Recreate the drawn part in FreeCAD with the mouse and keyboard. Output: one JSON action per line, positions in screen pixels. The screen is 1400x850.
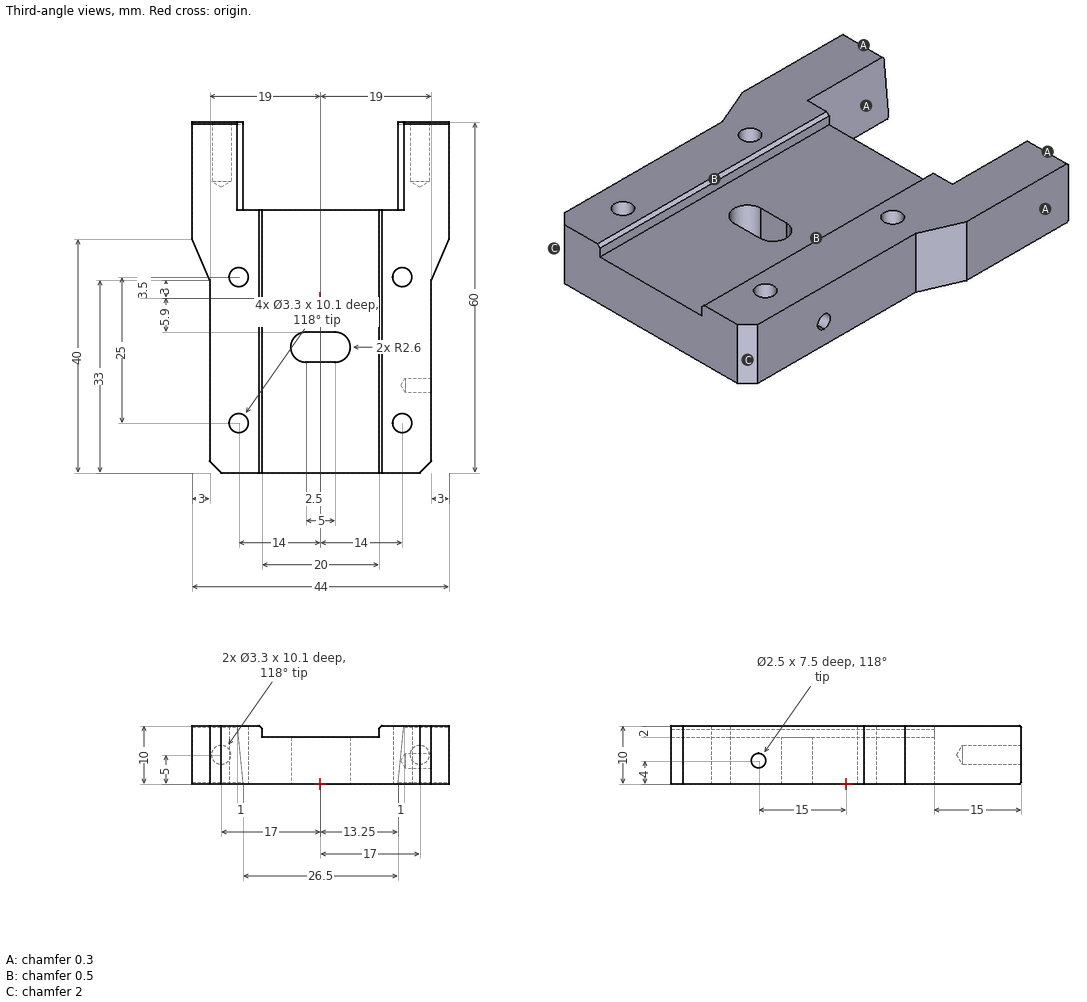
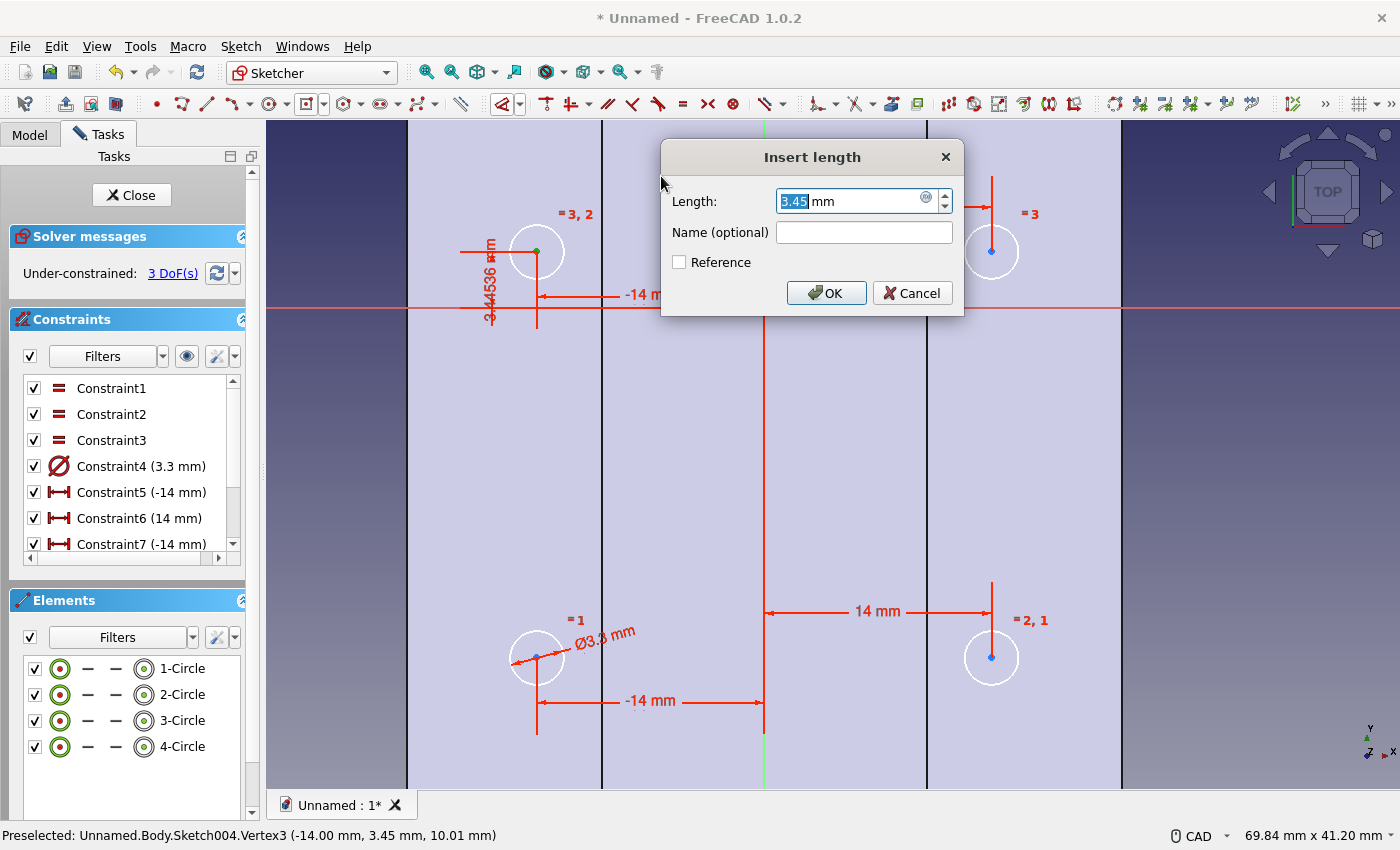
{"action": "type", "text": "3.5"}
{"action": "key", "text": "Return"}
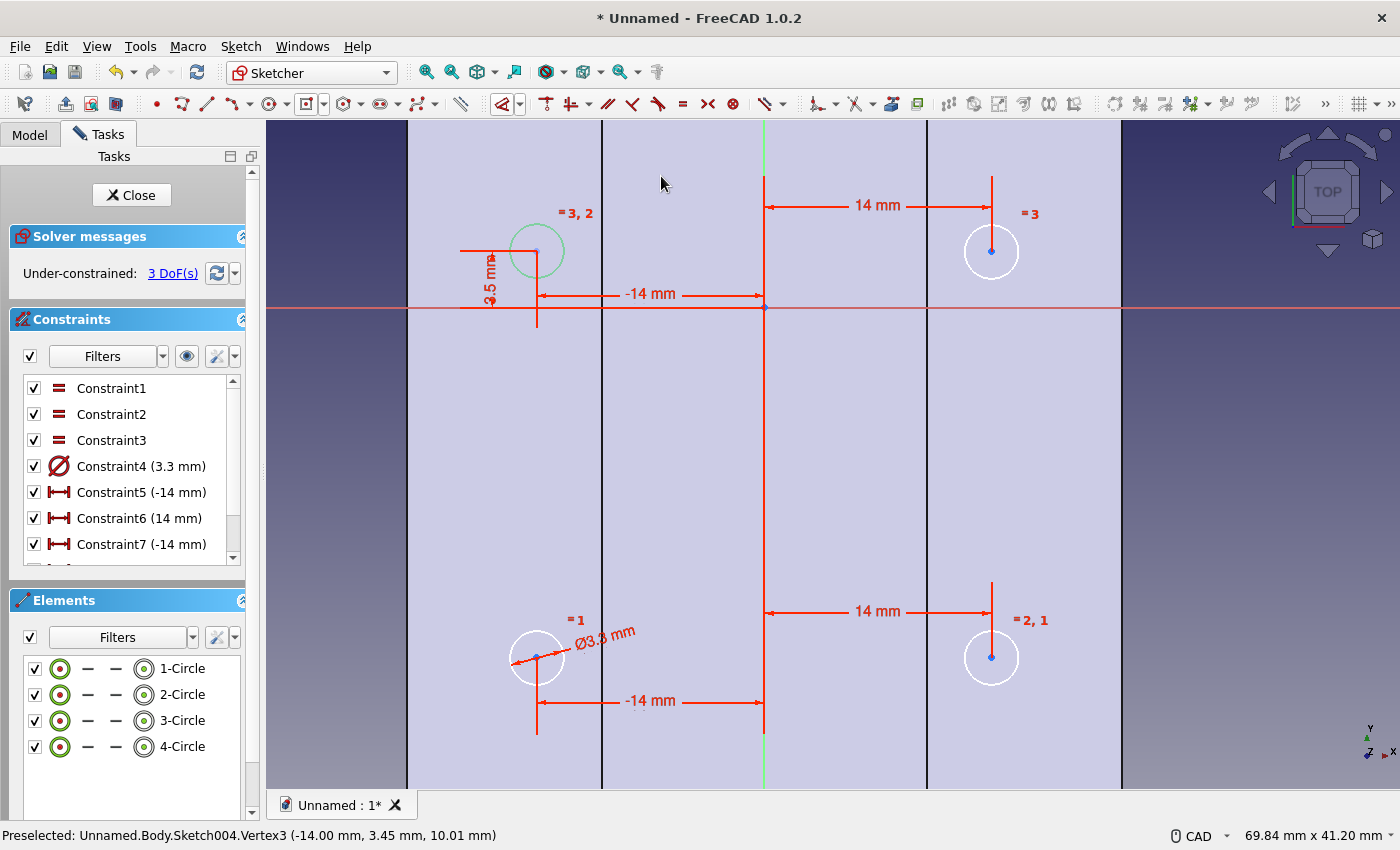
{"action": "left_click", "coordinate": [992, 252]}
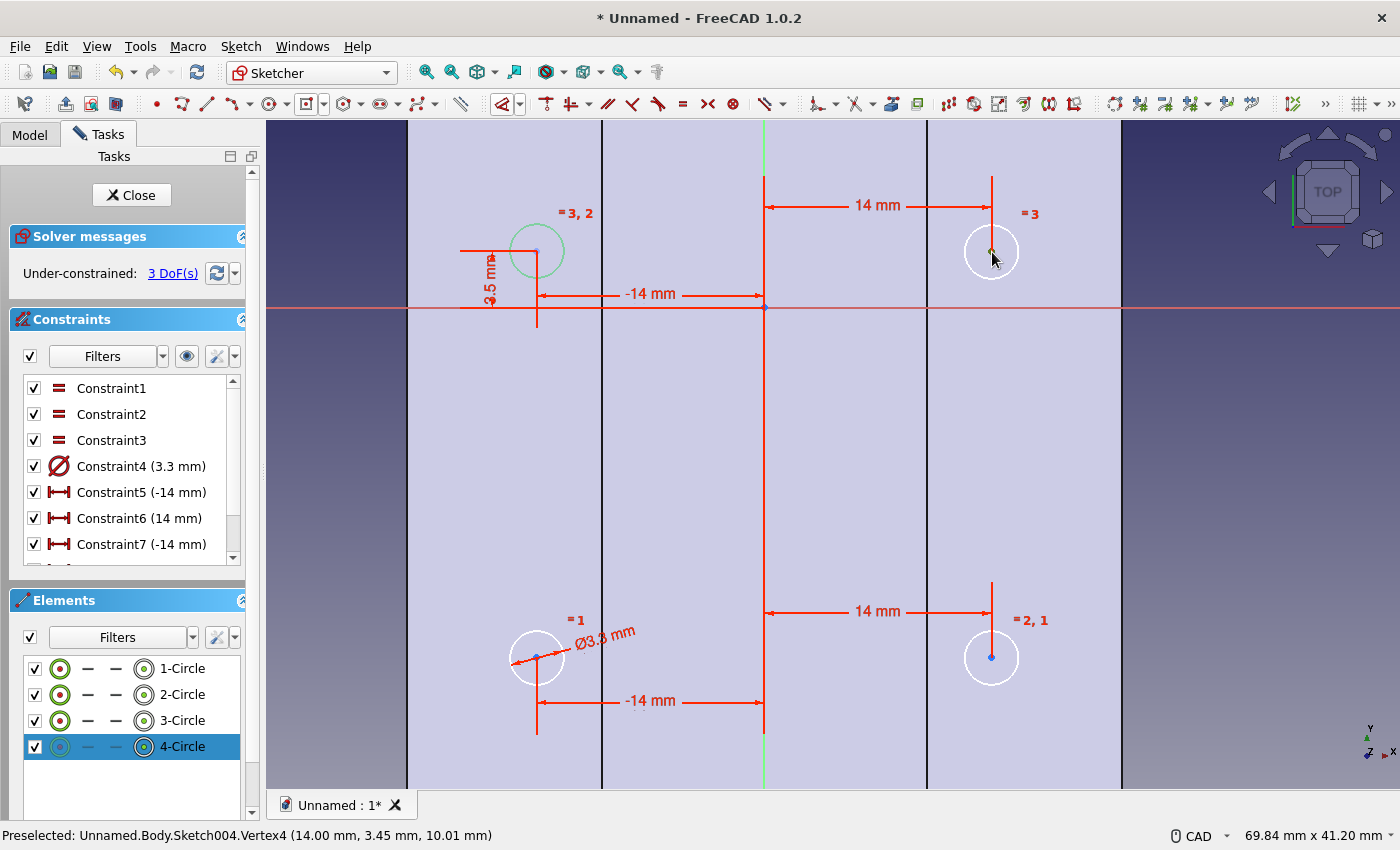
{"action": "key", "text": "i"}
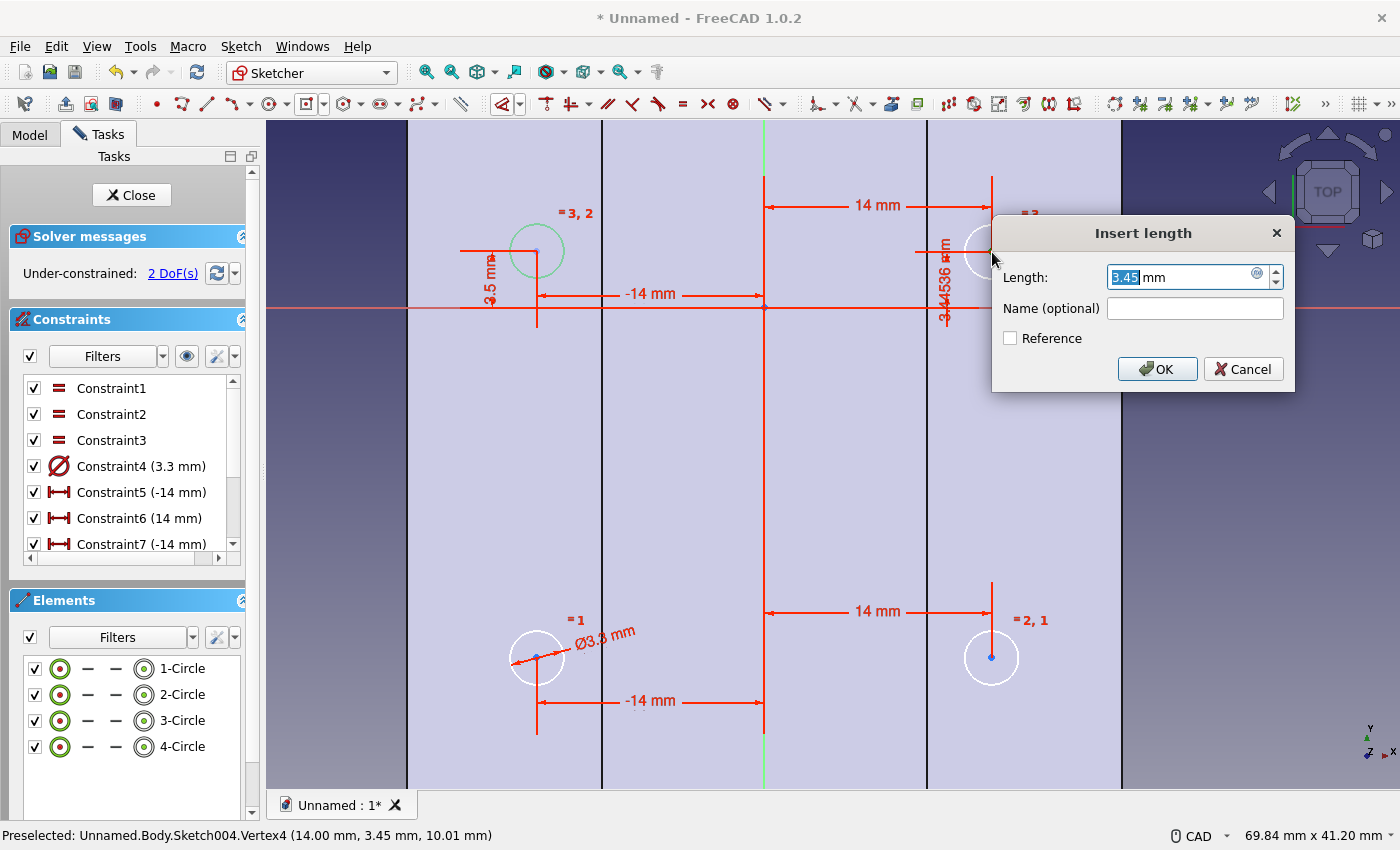
{"action": "type", "text": "3.5"}
{"action": "key", "text": "Return"}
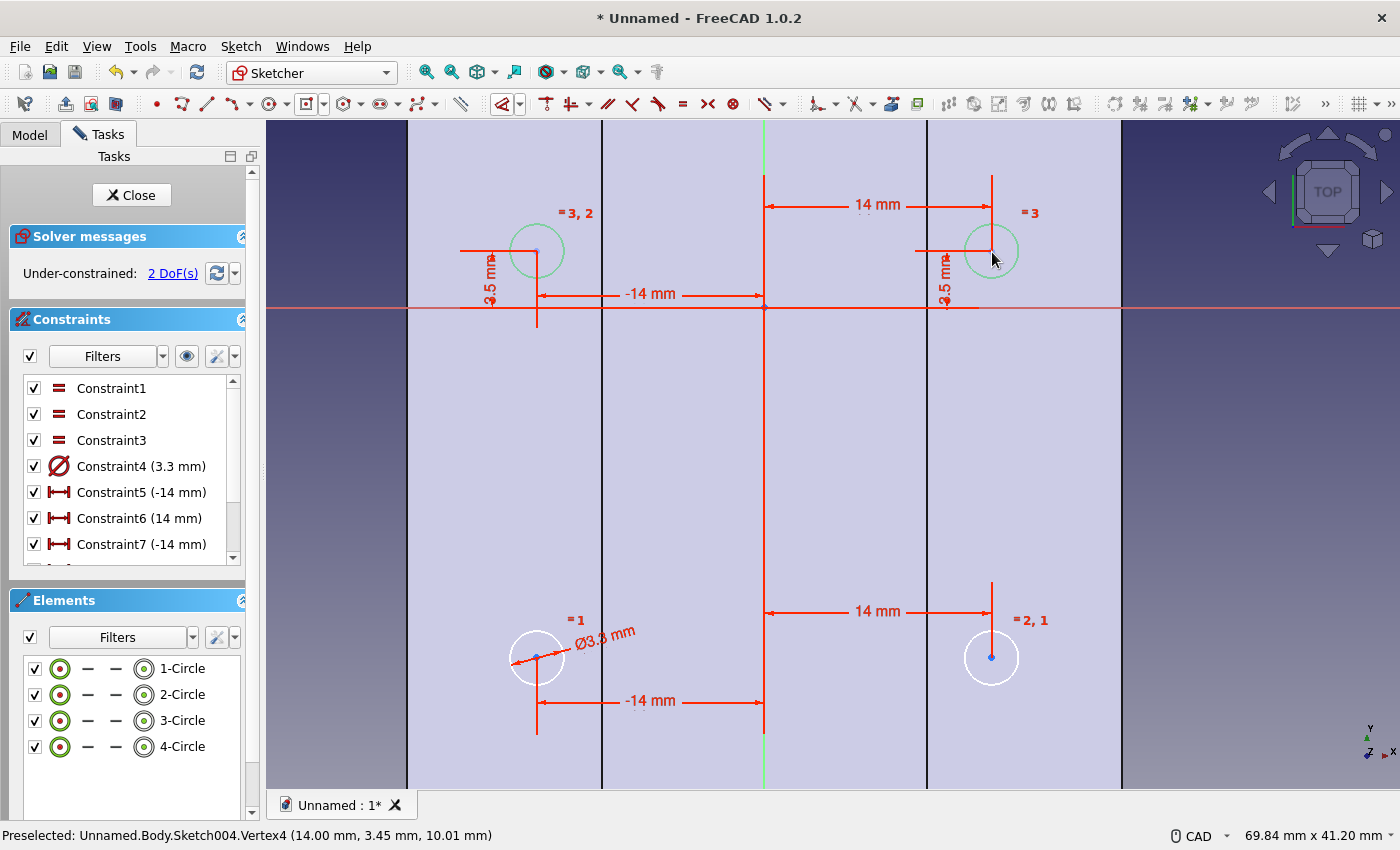
{"action": "left_click", "coordinate": [537, 658]}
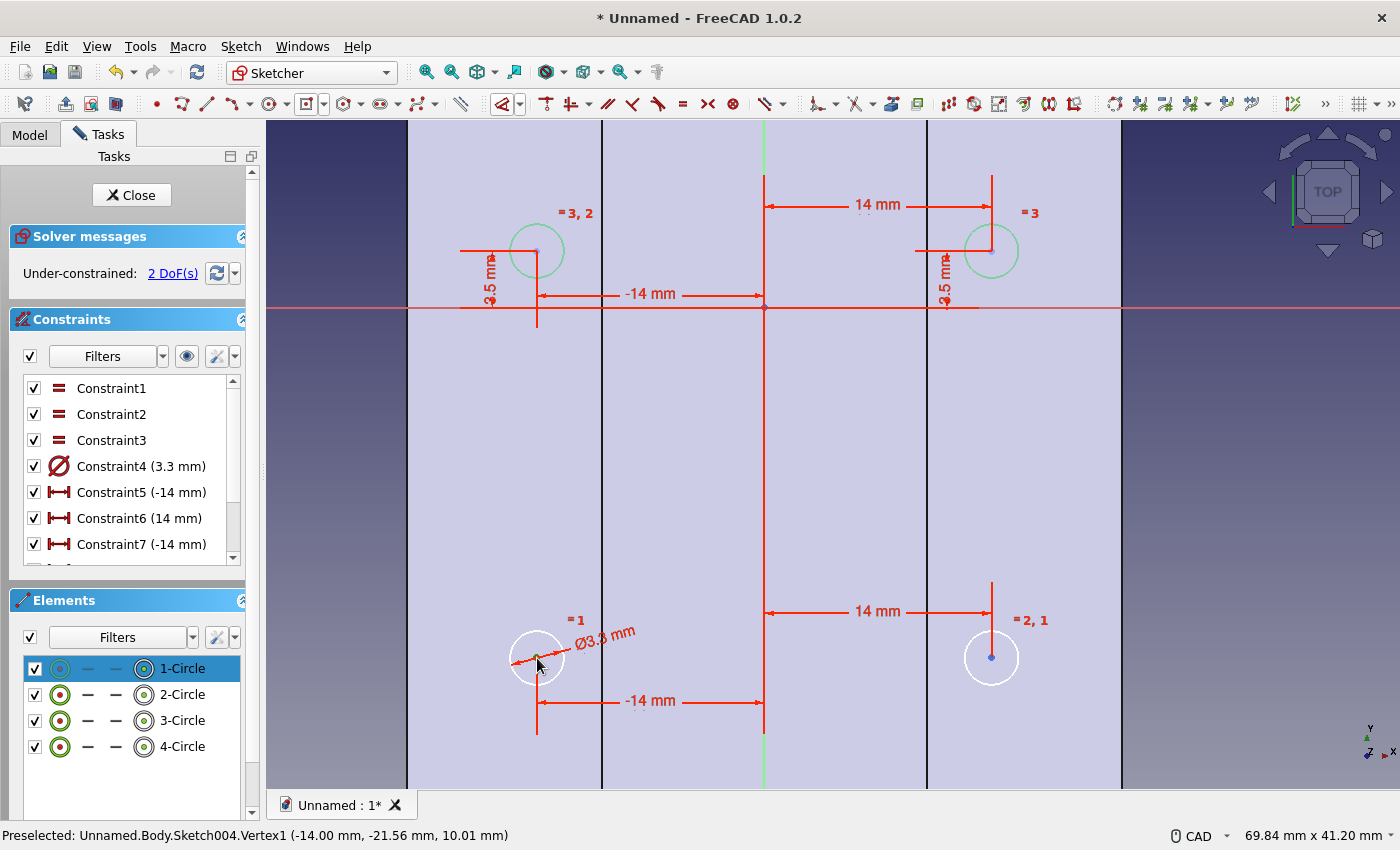
{"action": "left_click", "coordinate": [537, 251]}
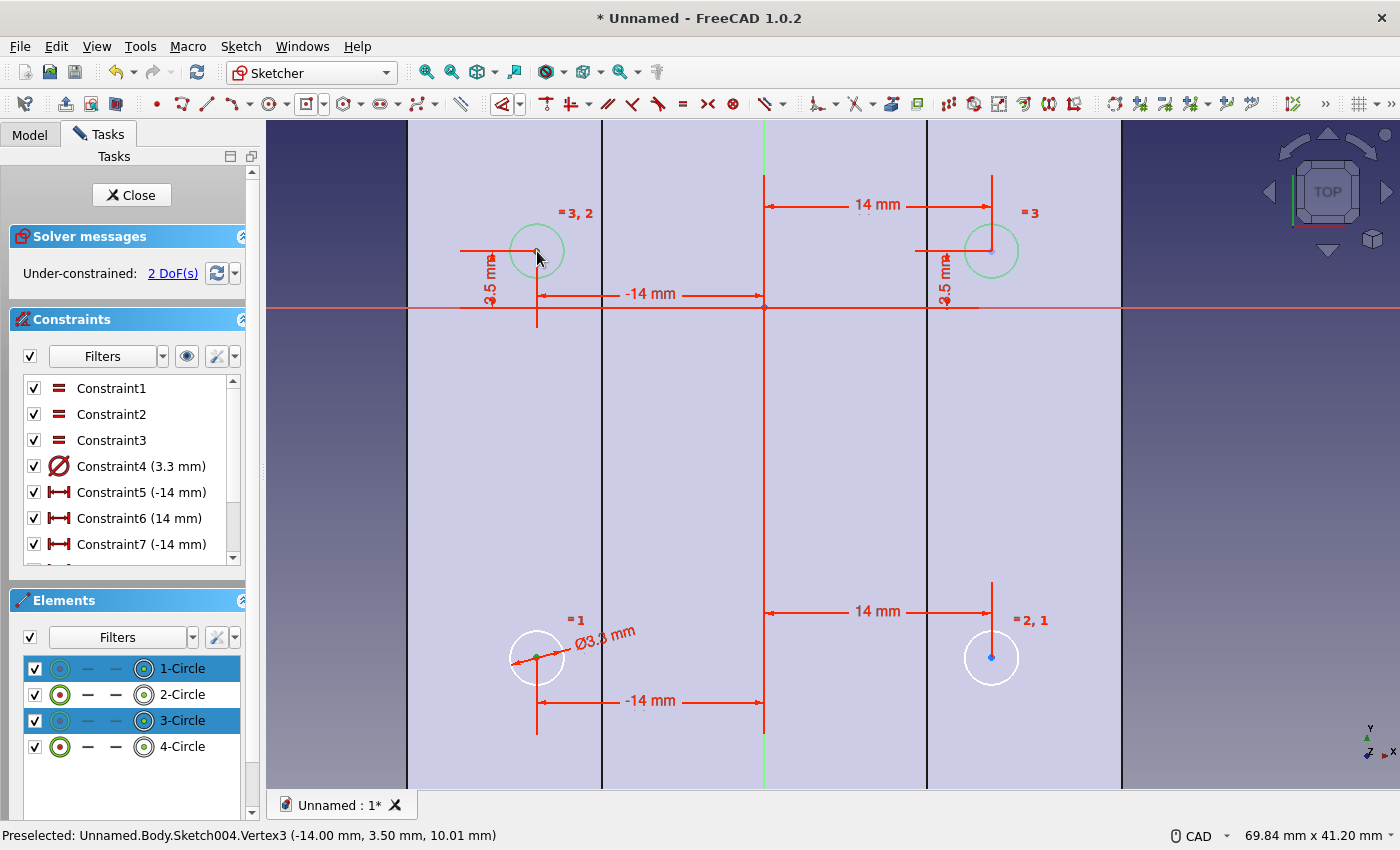
{"action": "key", "text": "i"}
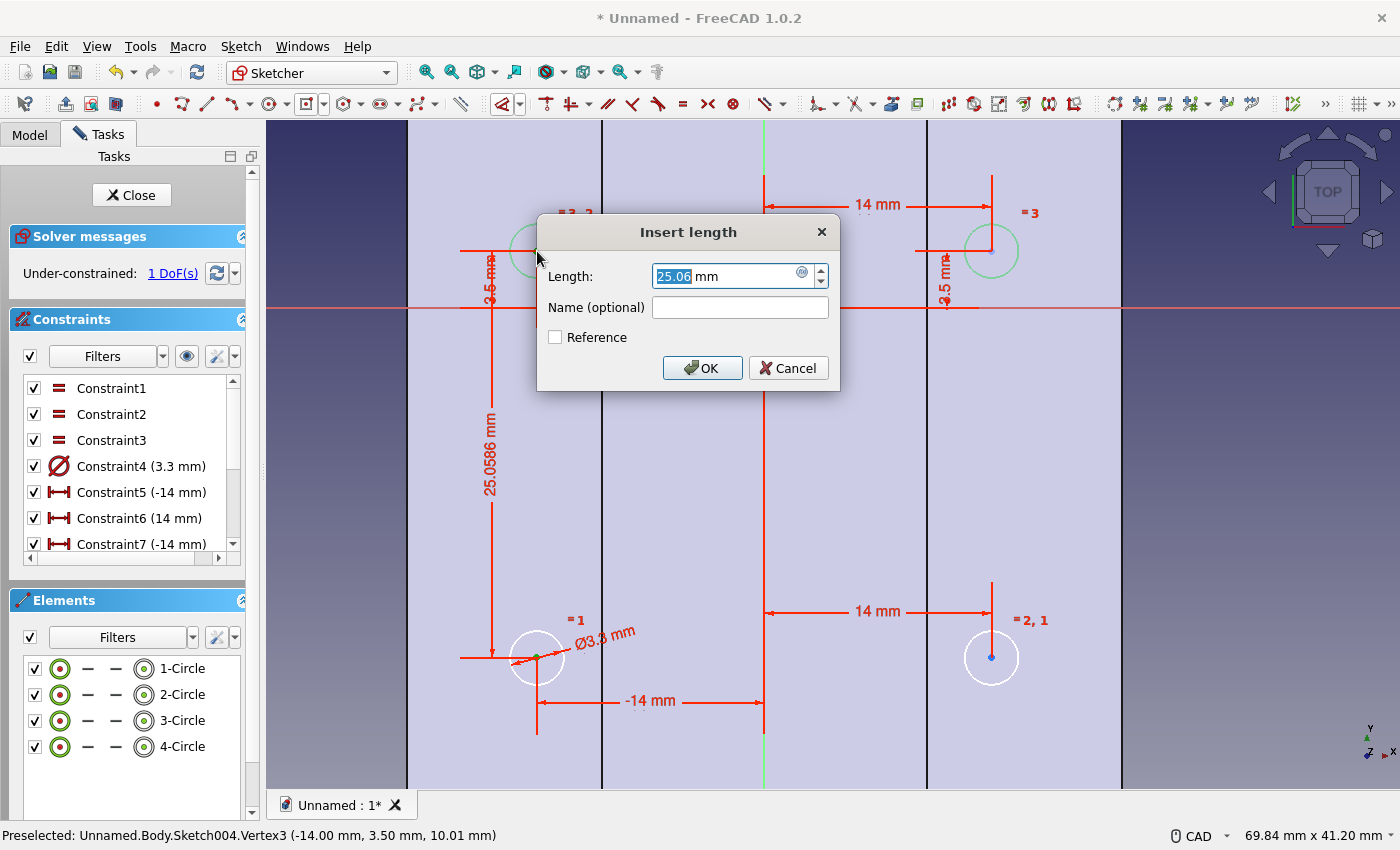
{"action": "type", "text": "25"}
{"action": "key", "text": "Return"}